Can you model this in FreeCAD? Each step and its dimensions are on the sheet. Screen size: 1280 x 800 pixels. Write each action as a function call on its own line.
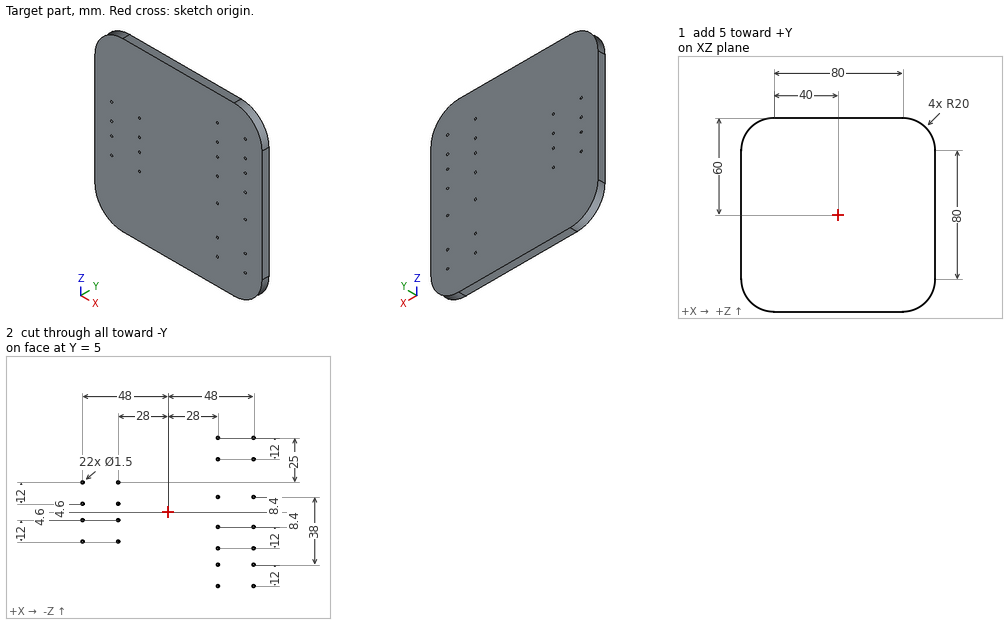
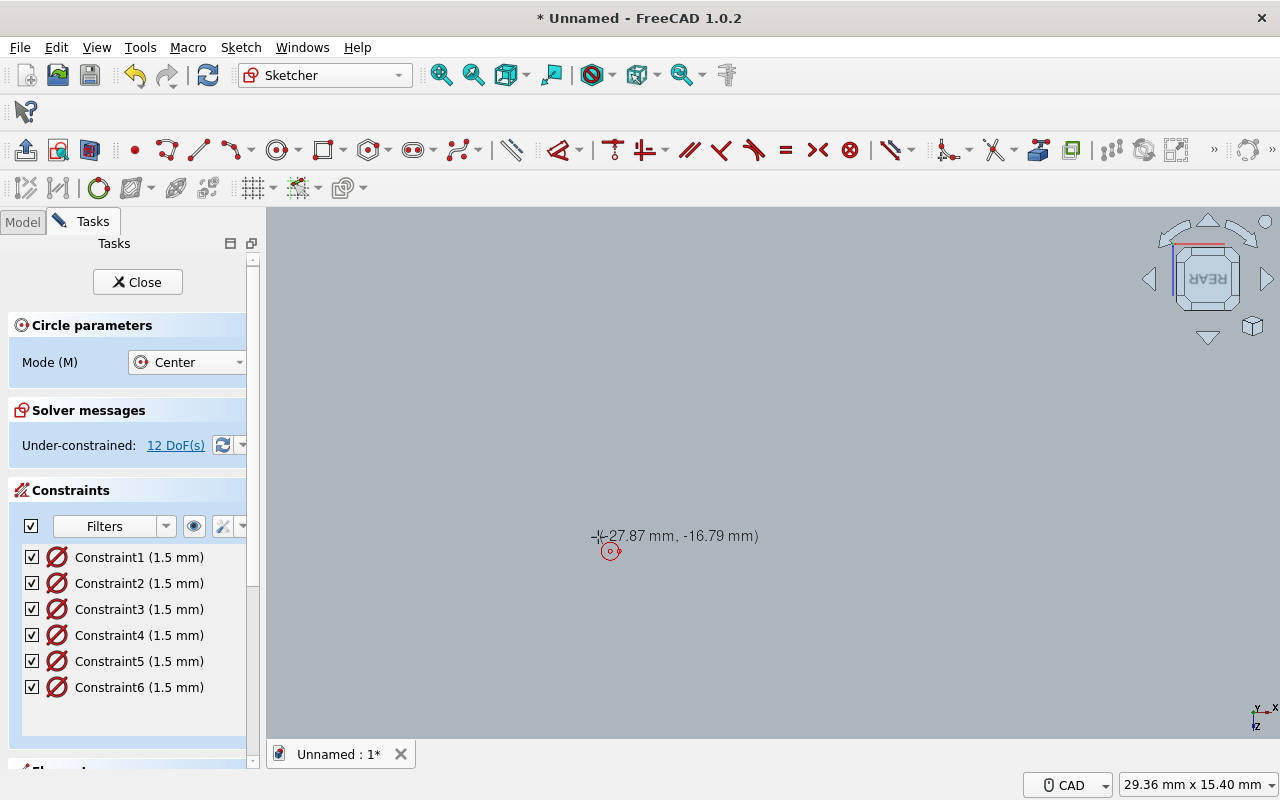
scroll(598, 537, down, 11)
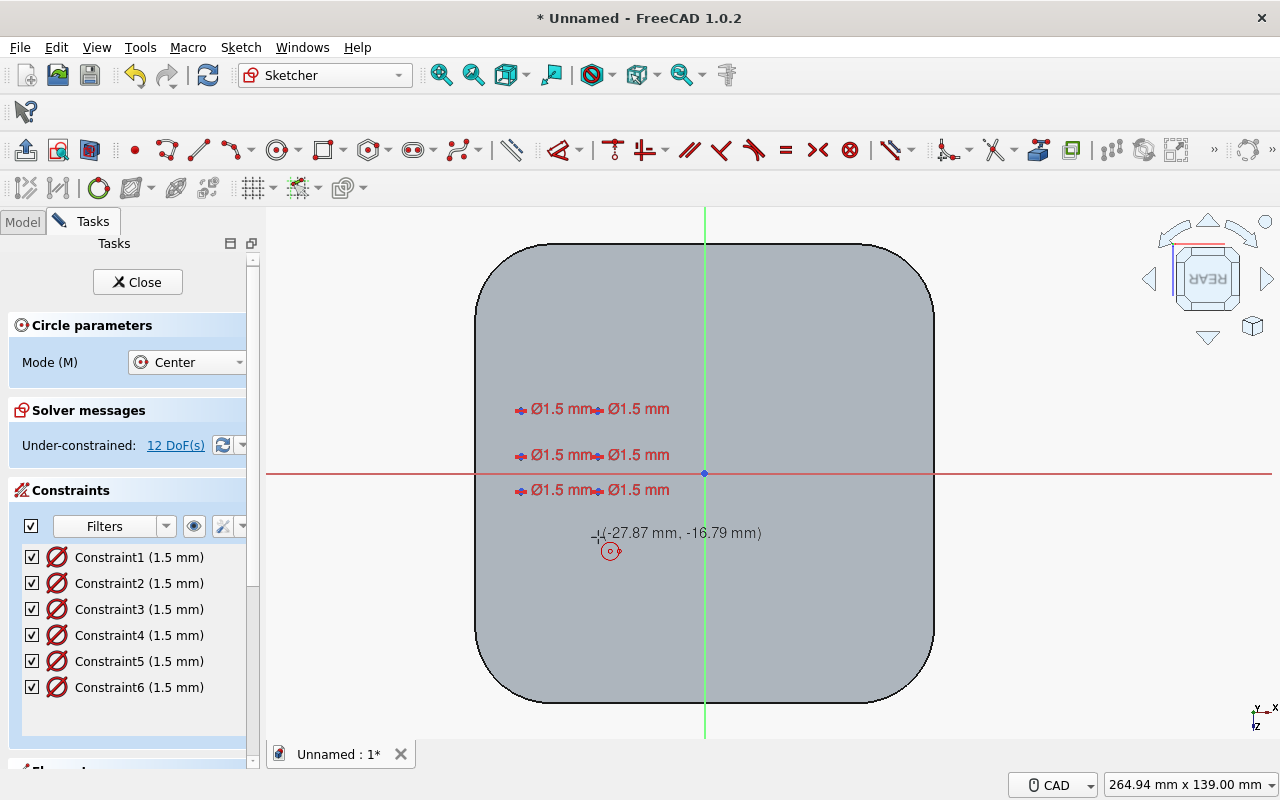
click(598, 537)
move(600, 535)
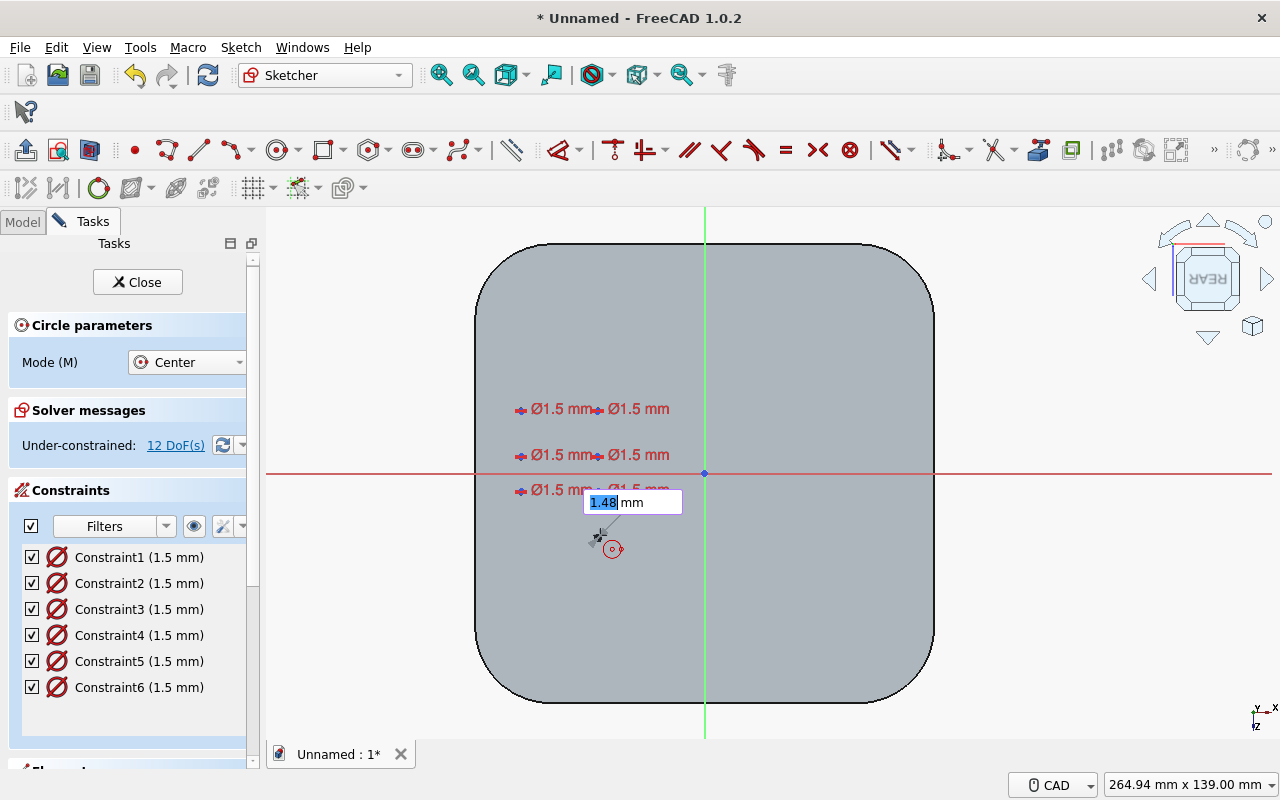
text(1.5)
key(Return)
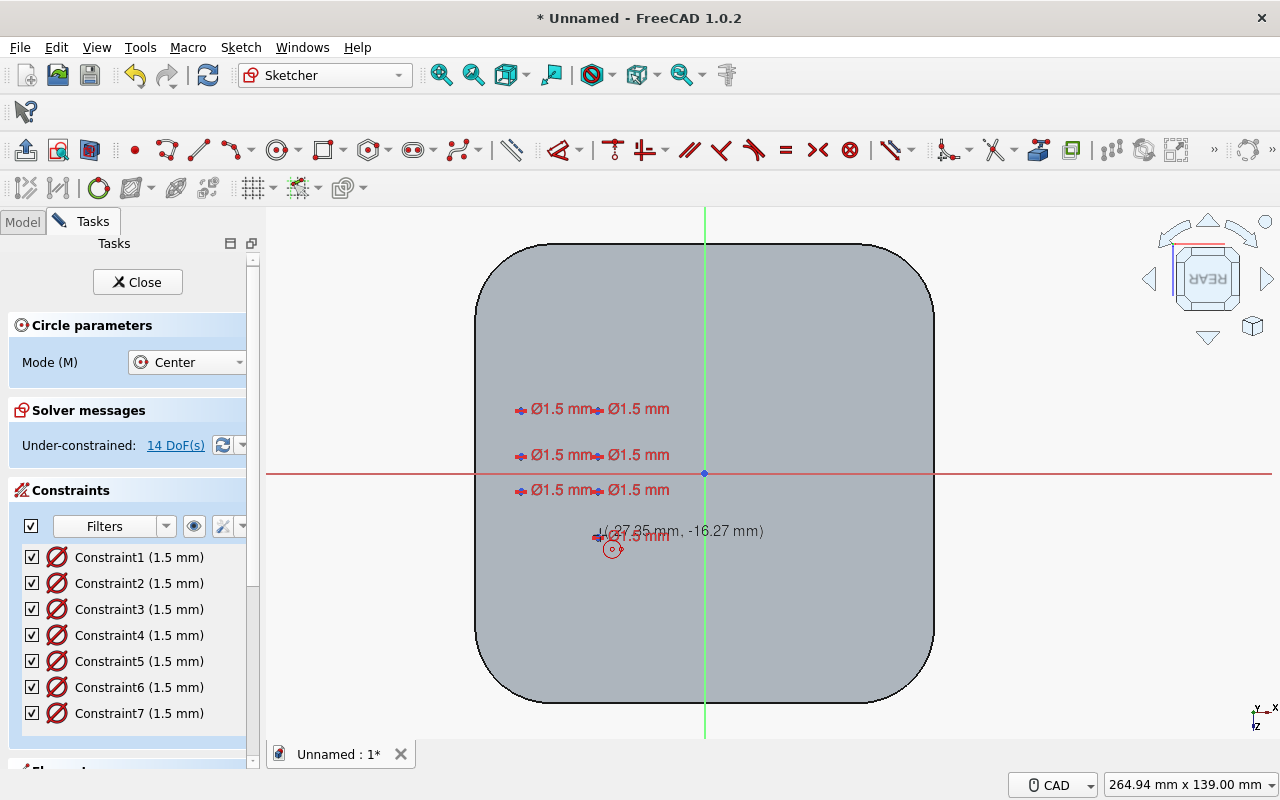
scroll(521, 537, up, 11)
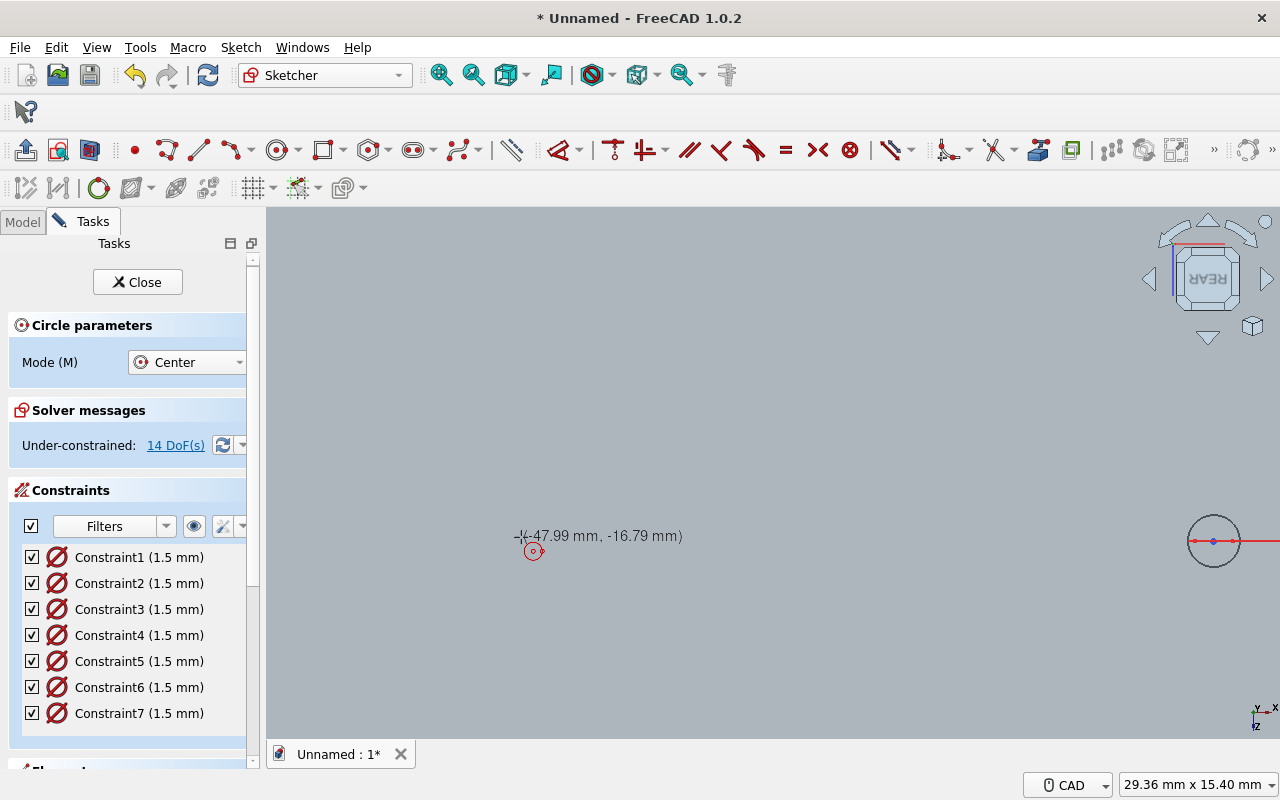
scroll(521, 537, down, 11)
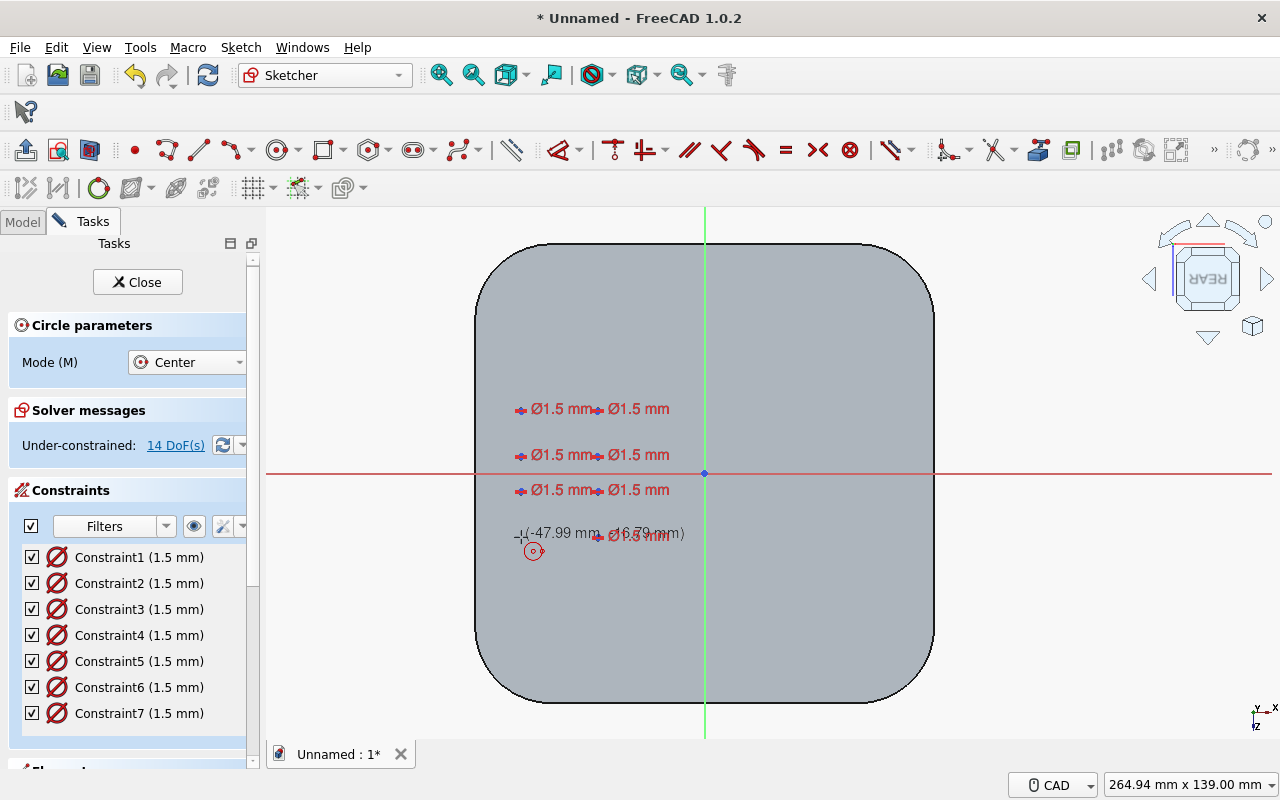
click(521, 537)
move(523, 535)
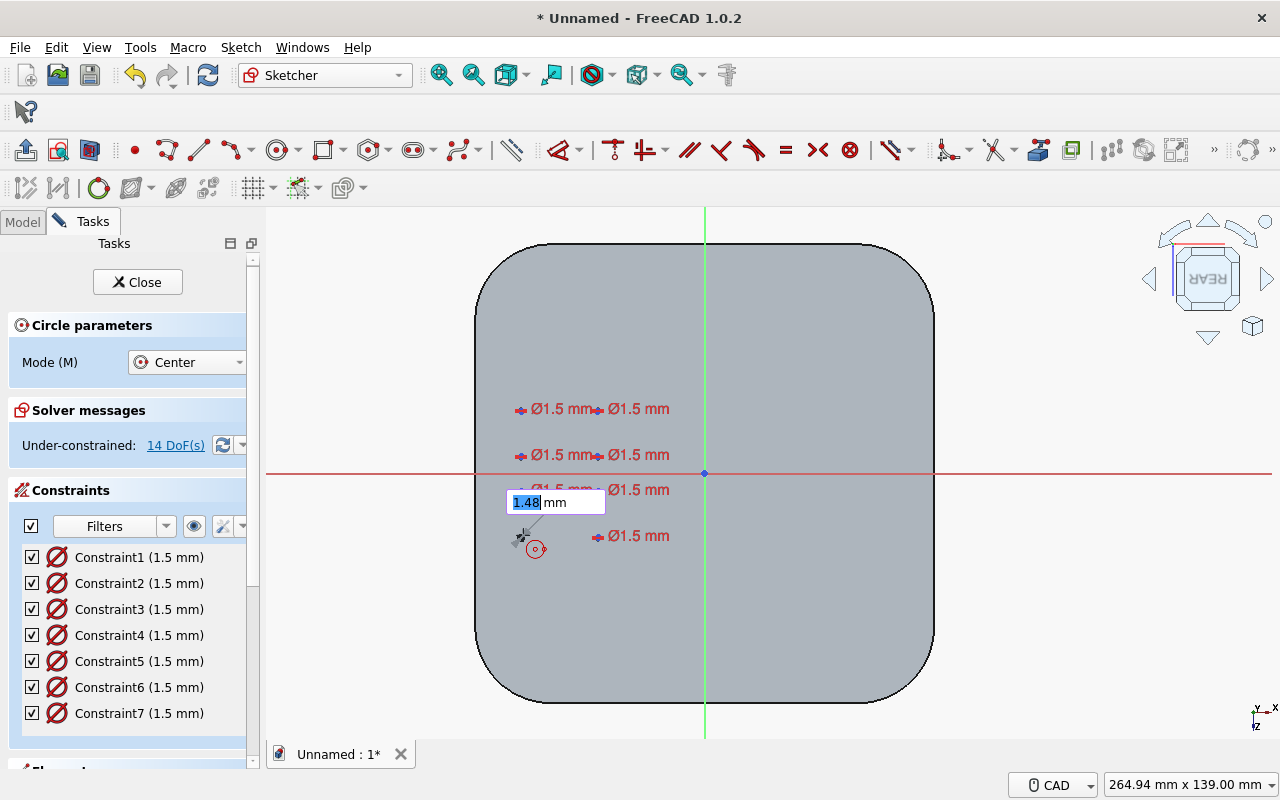
text(1.5)
key(Return)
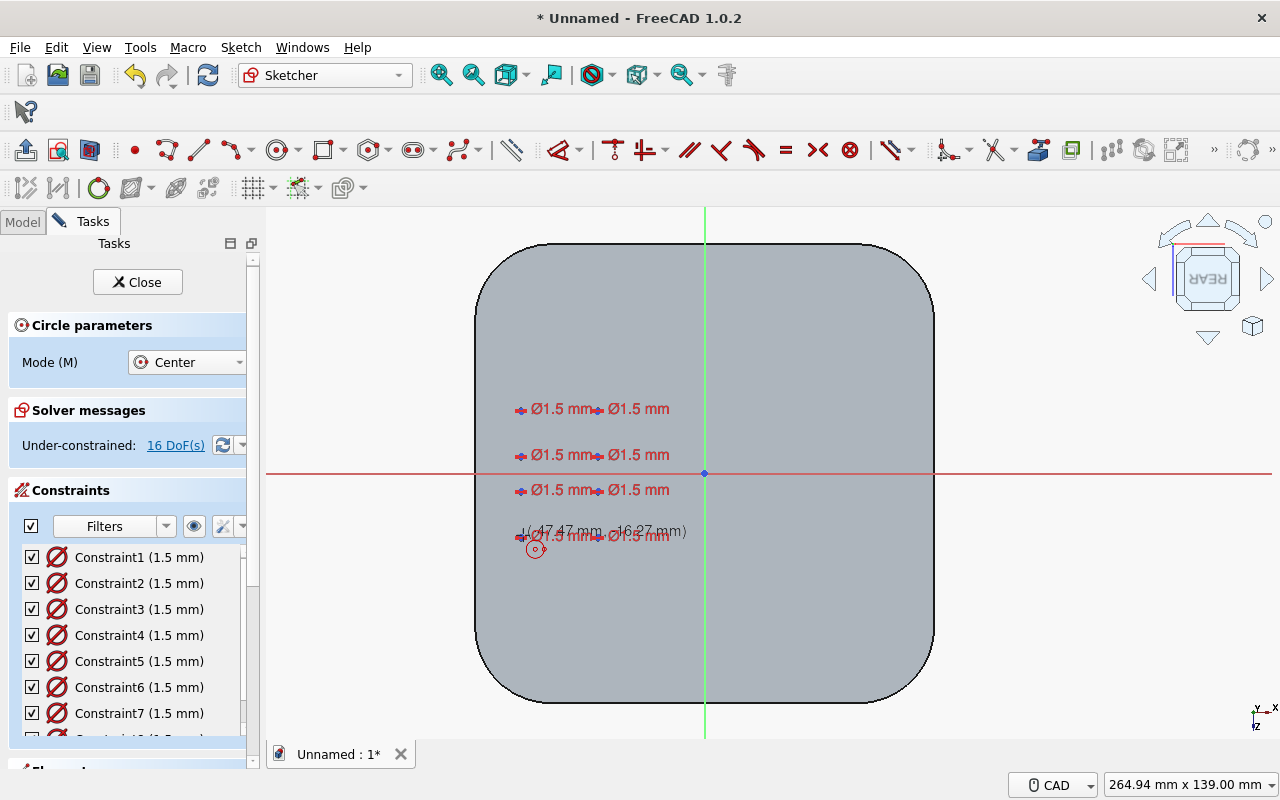
scroll(812, 315, up, 11)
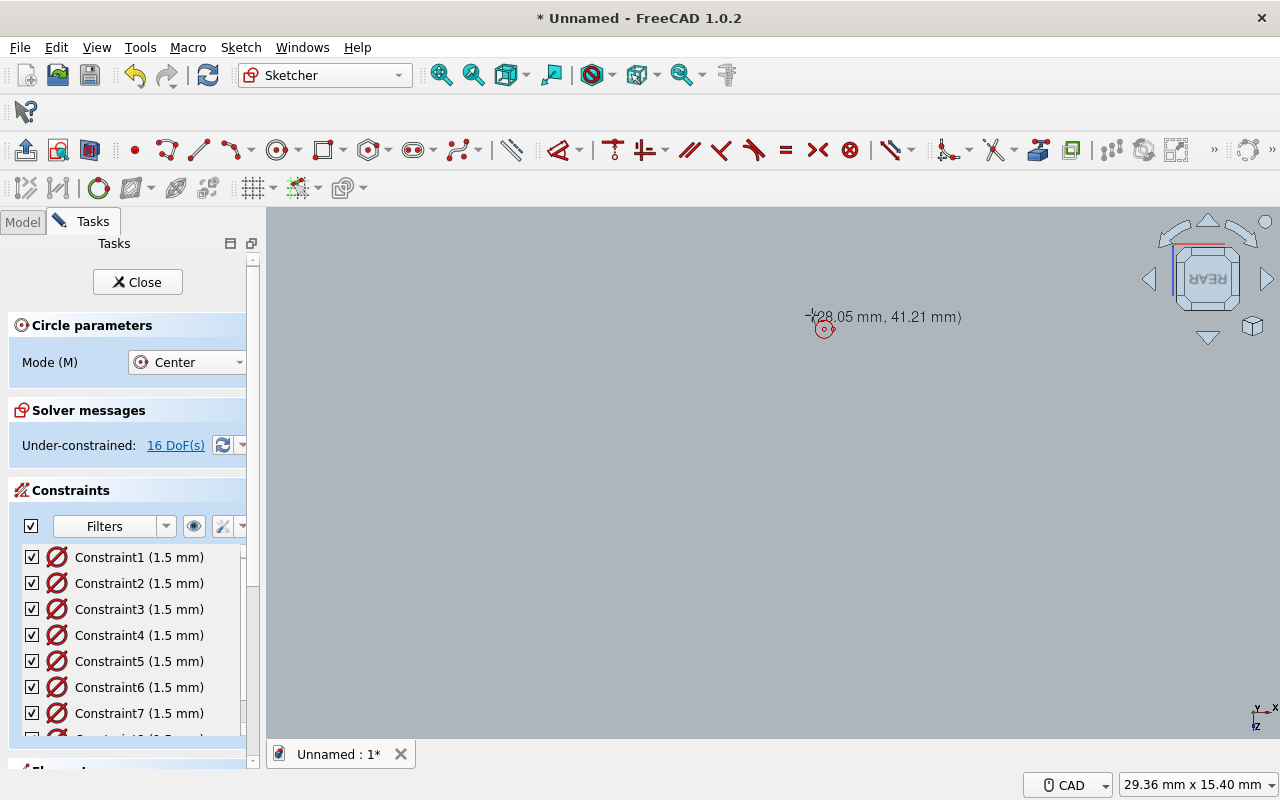
scroll(812, 314, down, 11)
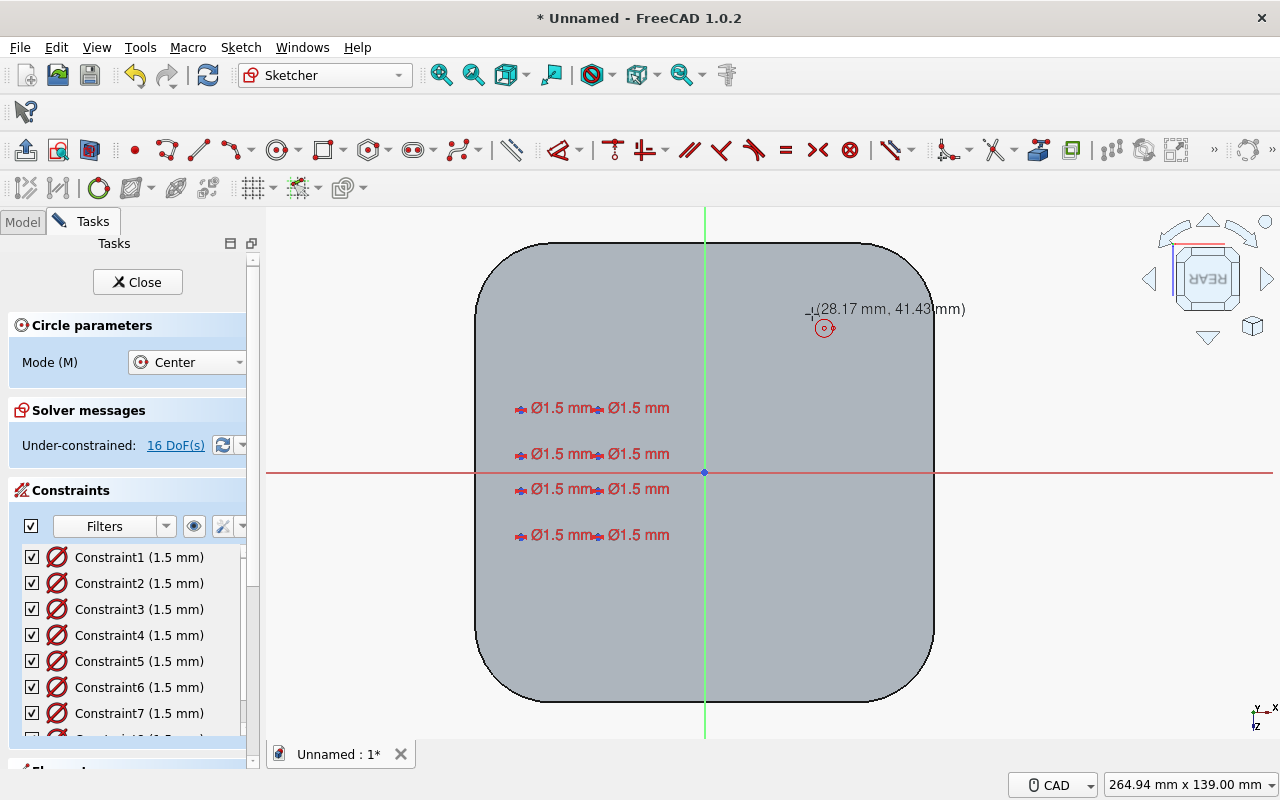
click(812, 314)
move(814, 312)